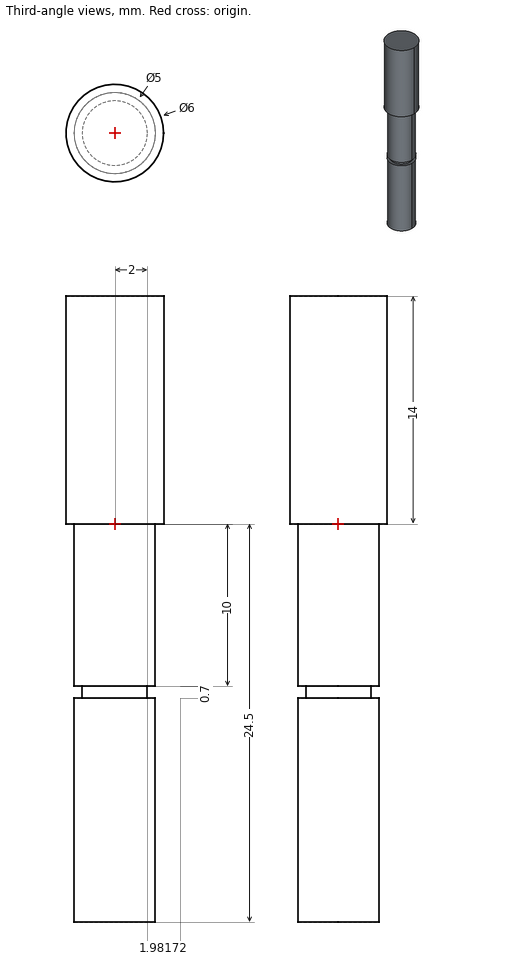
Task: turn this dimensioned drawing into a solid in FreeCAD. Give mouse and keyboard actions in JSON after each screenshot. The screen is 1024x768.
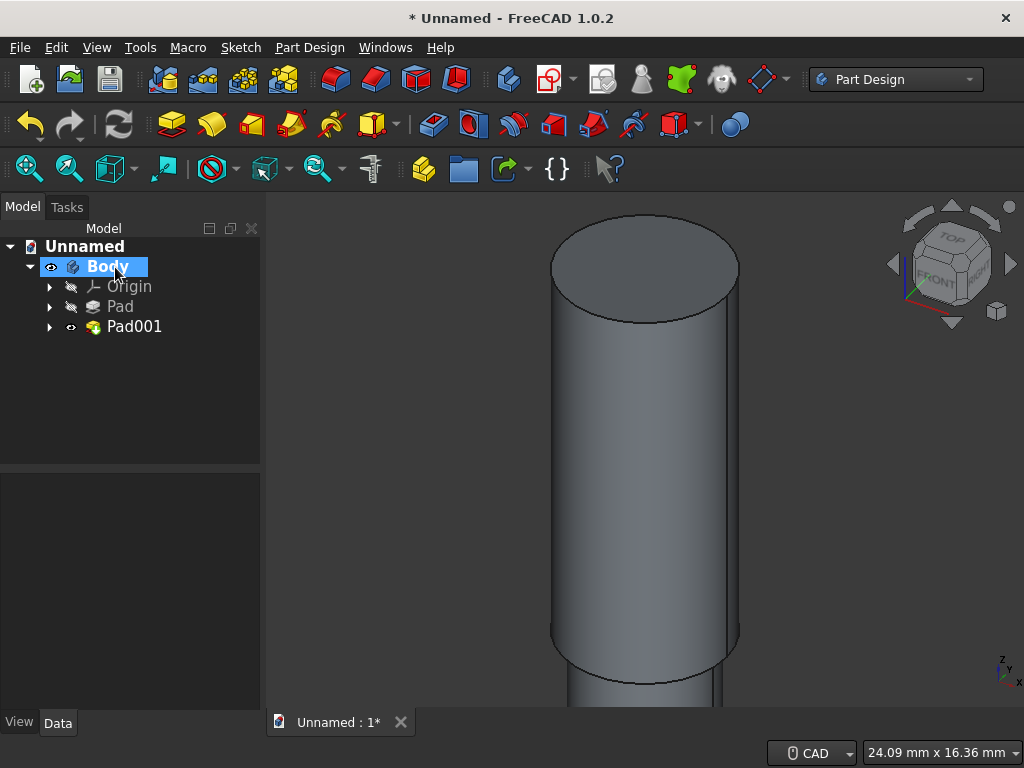
{"action": "left_click", "coordinate": [30, 170]}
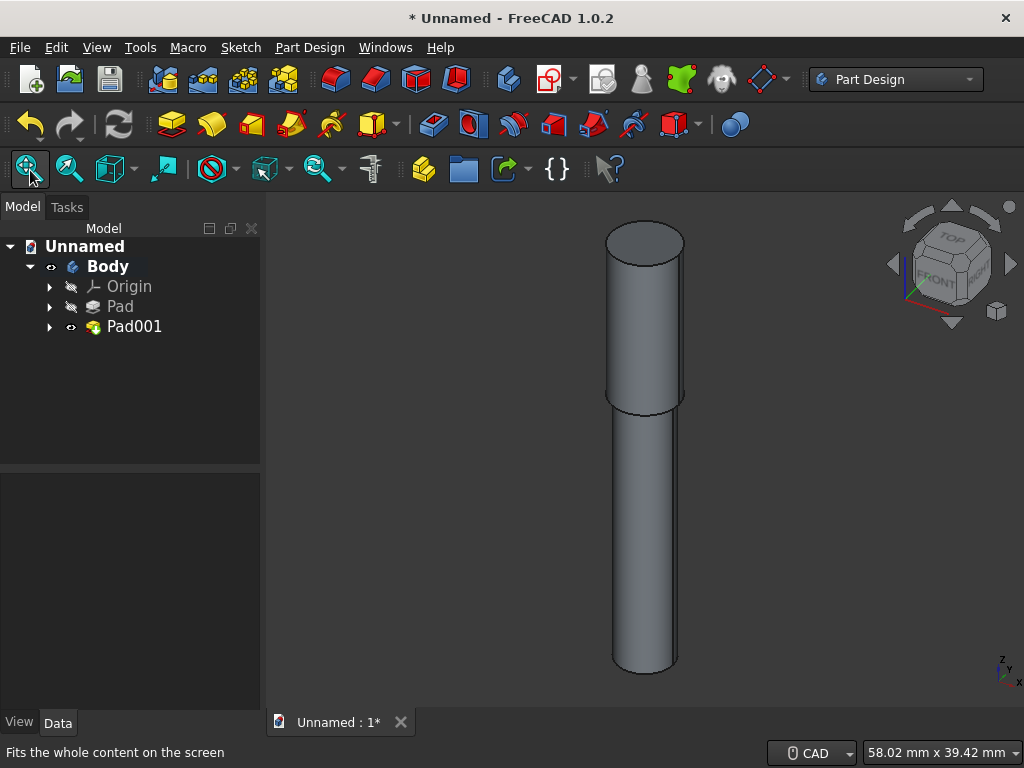
{"action": "left_click", "coordinate": [550, 80]}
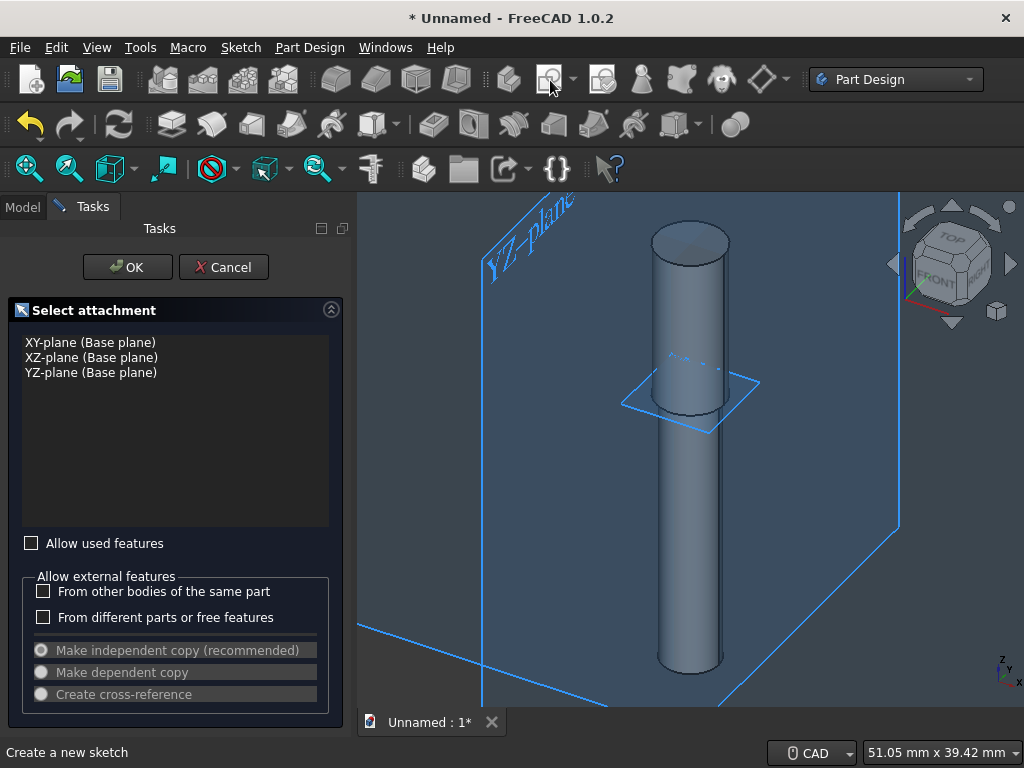
{"action": "left_click", "coordinate": [82, 358]}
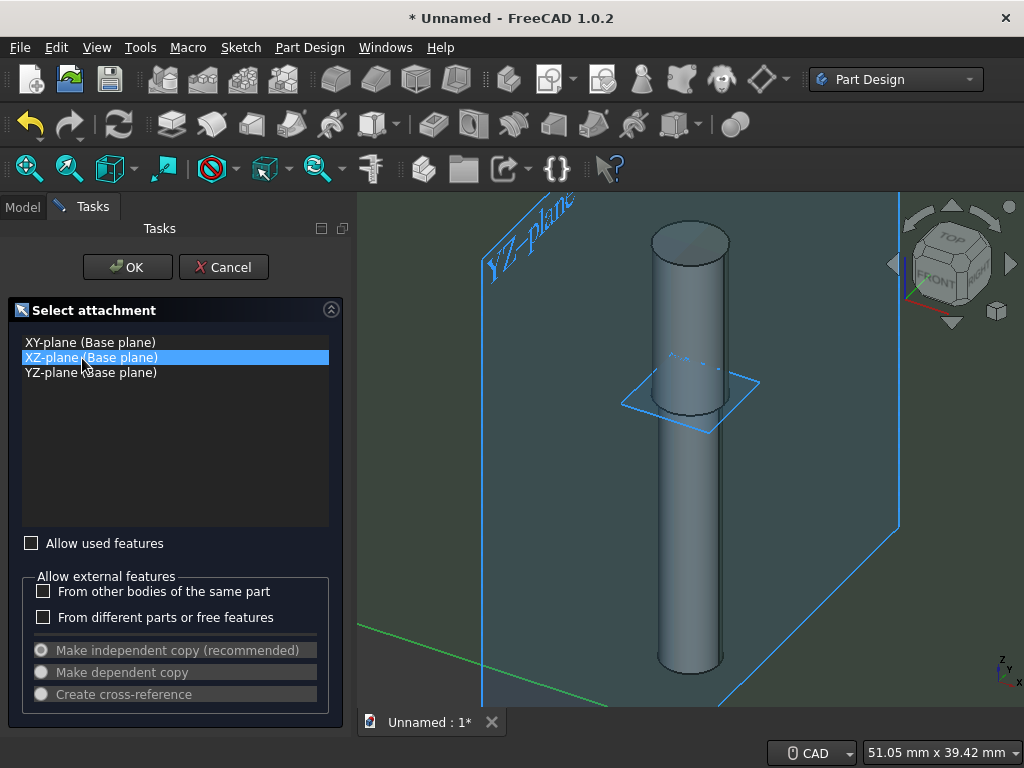
{"action": "left_click", "coordinate": [128, 267]}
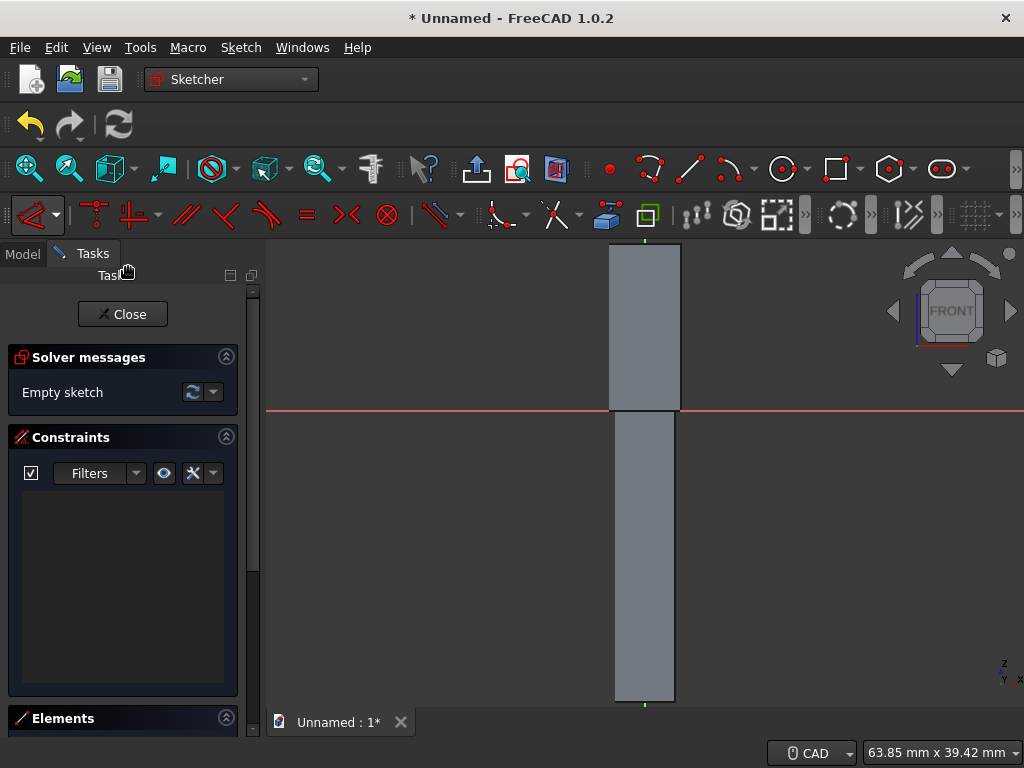
{"action": "left_click", "coordinate": [558, 170]}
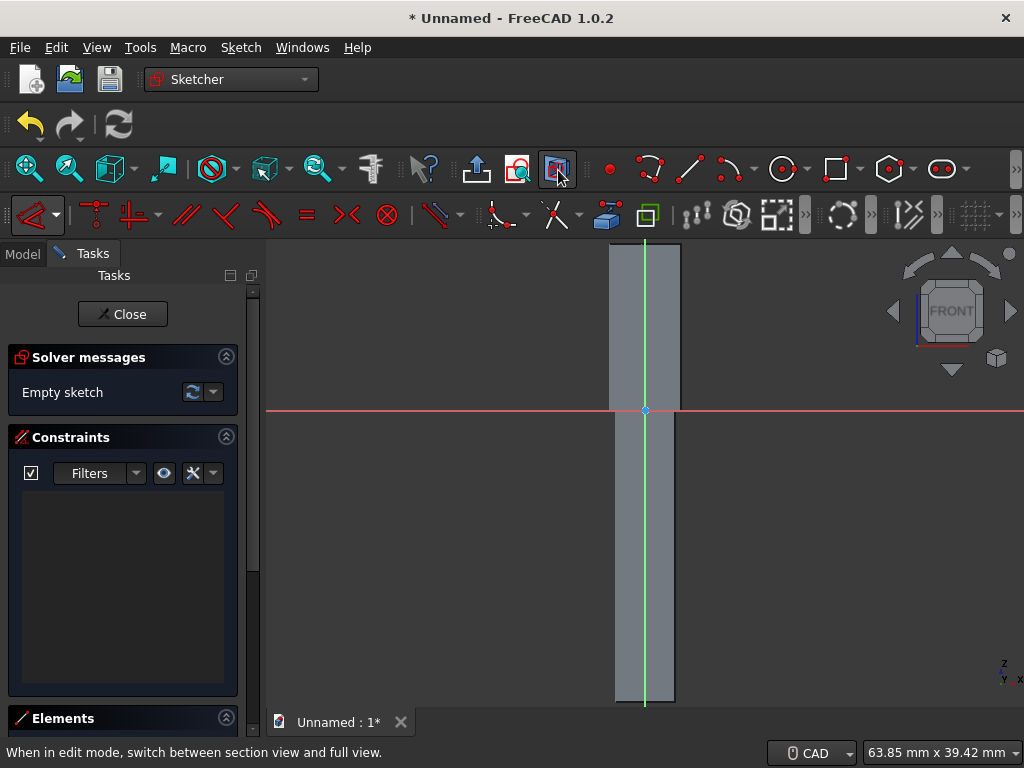
{"action": "scroll", "coordinate": [687, 537], "scroll_direction": "up", "scroll_amount": 14}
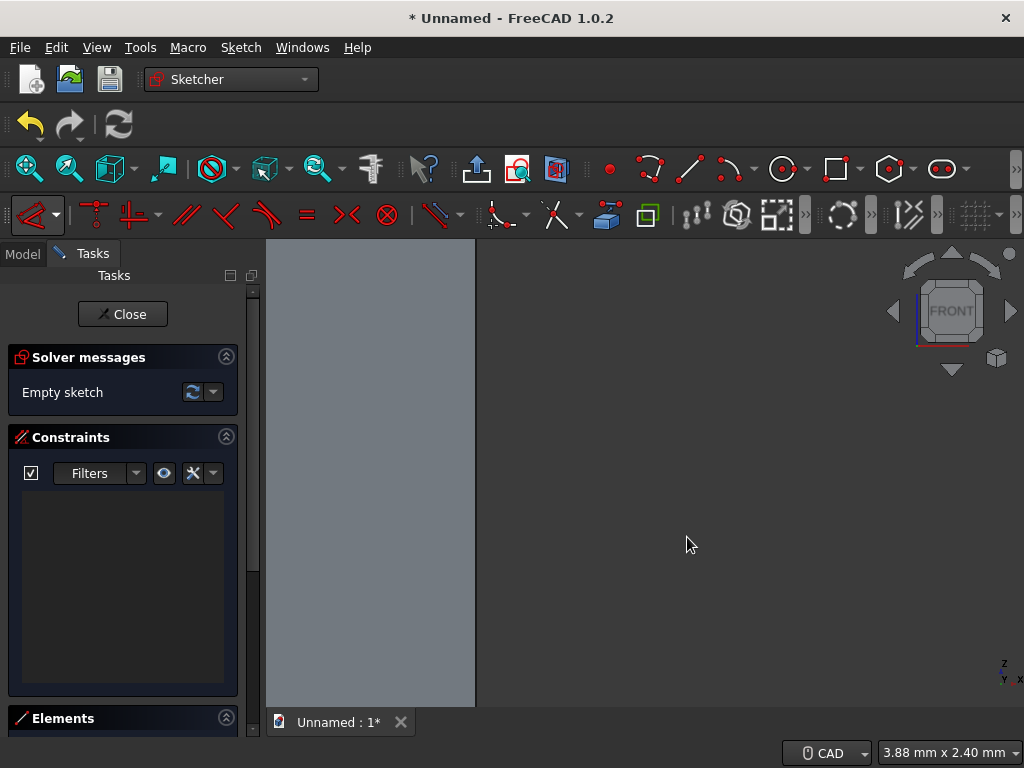
{"action": "left_click", "coordinate": [836, 170]}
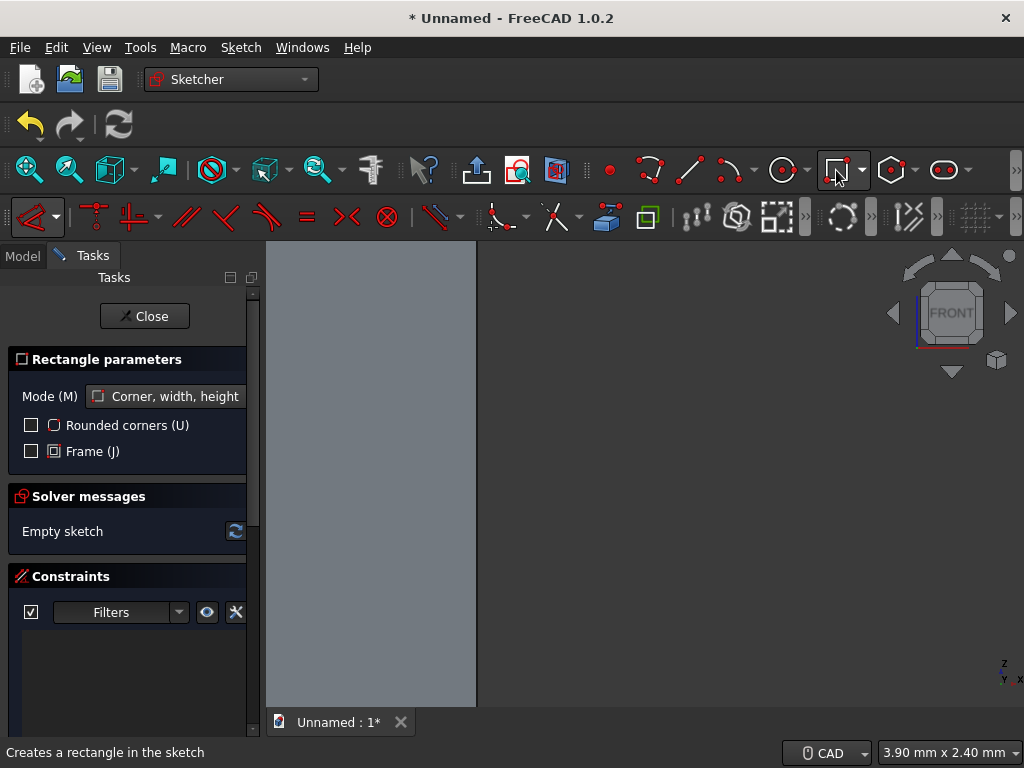
{"action": "left_click", "coordinate": [379, 403]}
{"action": "mouse_move", "coordinate": [765, 539]}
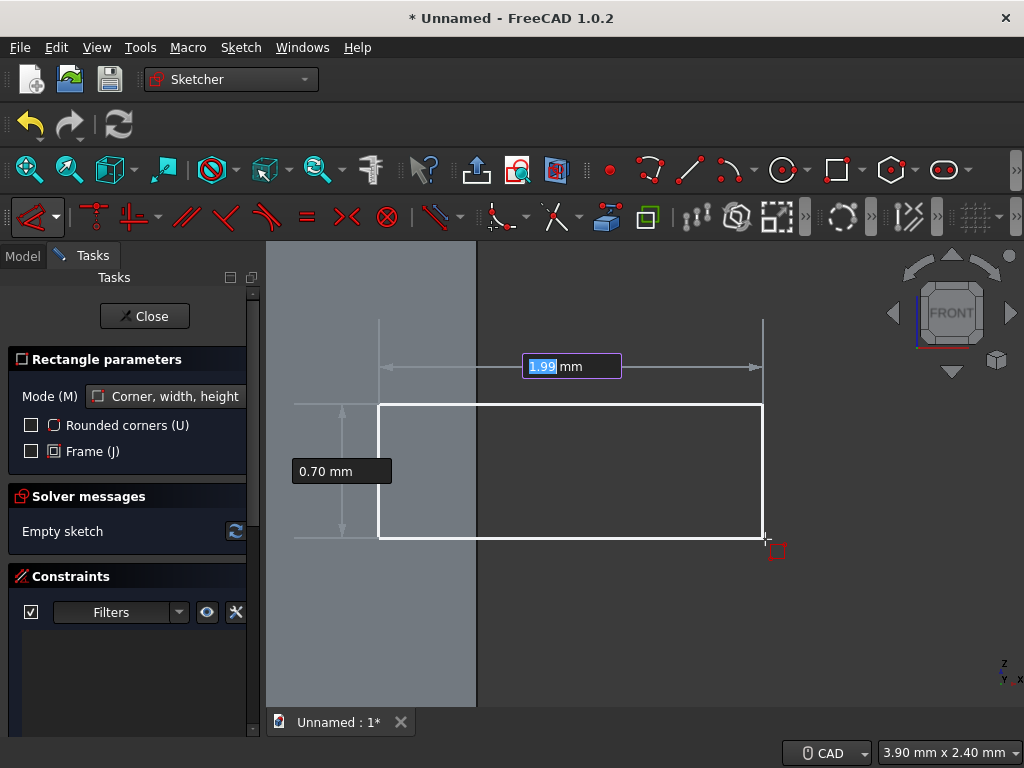
{"action": "type", "text": "1.98172"}
{"action": "key", "text": "Tab"}
{"action": "type", "text": "0.7"}
{"action": "key", "text": "Return"}
{"action": "key", "text": "Escape"}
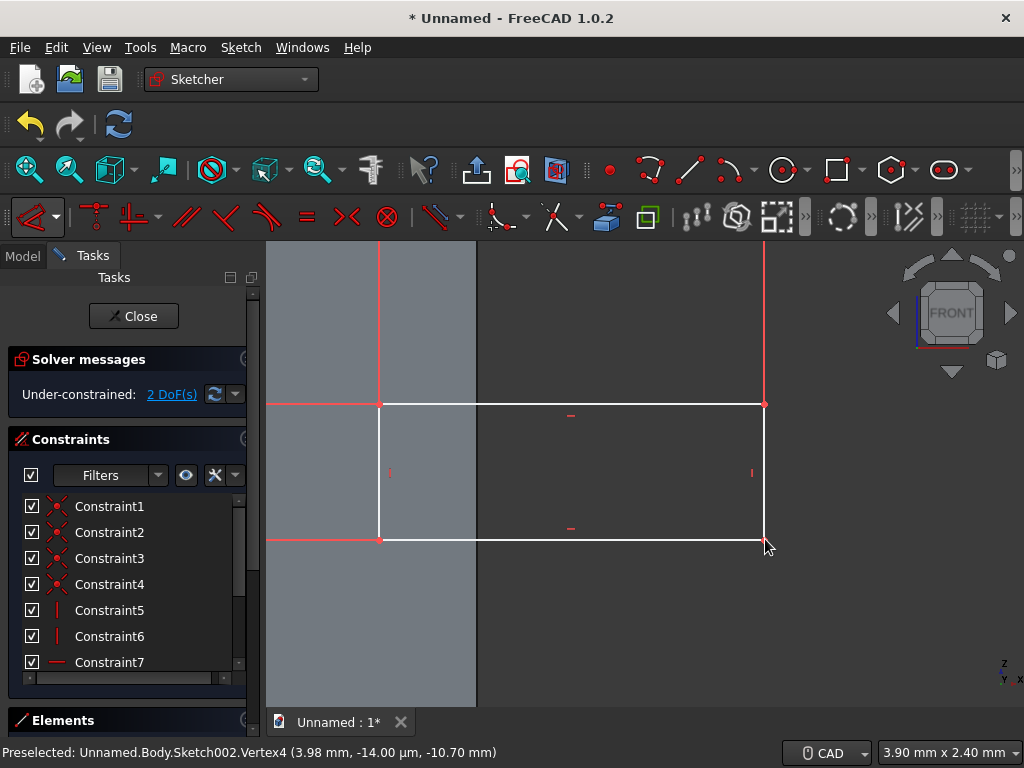
{"action": "left_click", "coordinate": [32, 218]}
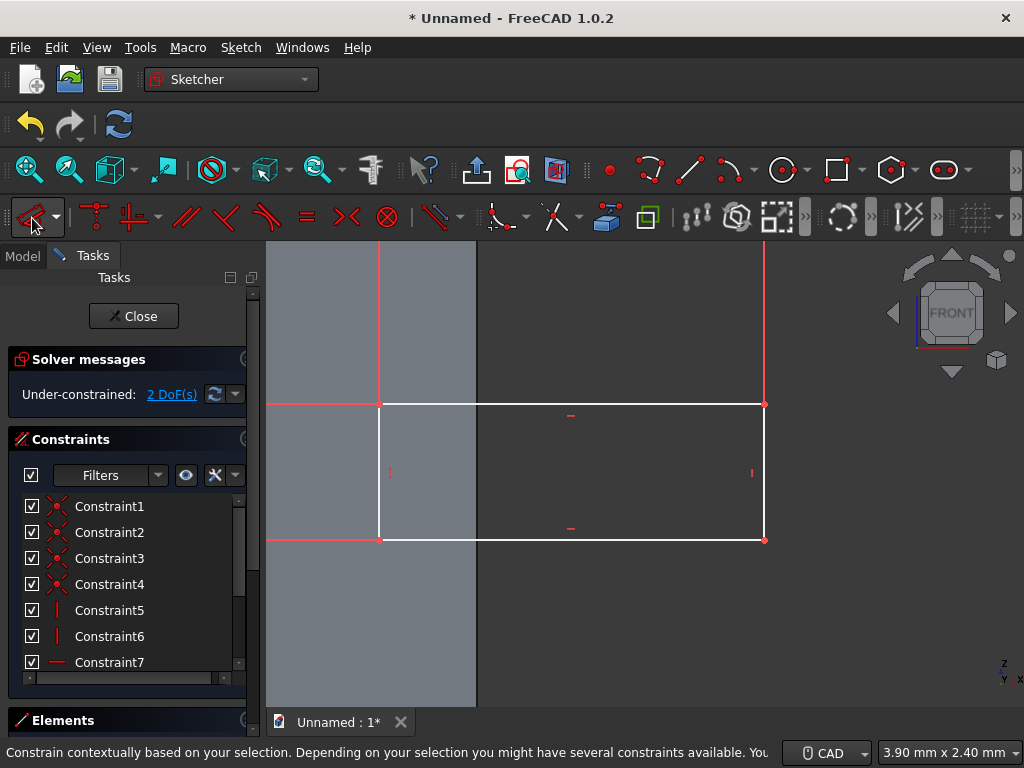
{"action": "left_click", "coordinate": [379, 404]}
{"action": "left_click", "coordinate": [336, 438]}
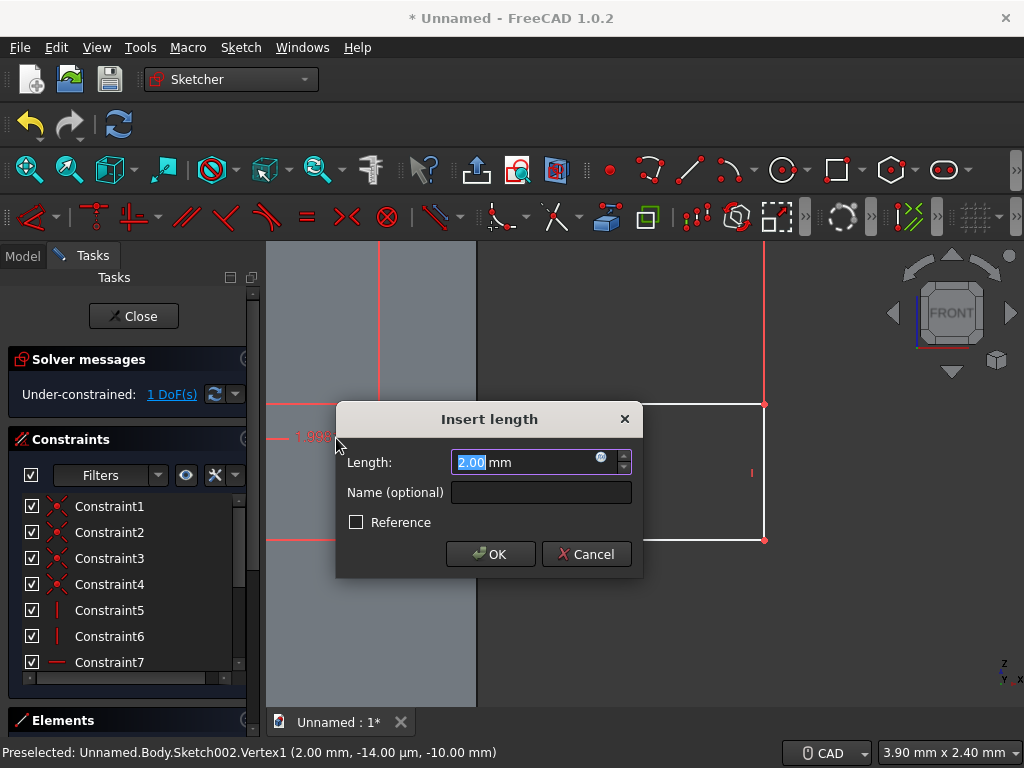
{"action": "type", "text": "2"}
{"action": "key", "text": "Return"}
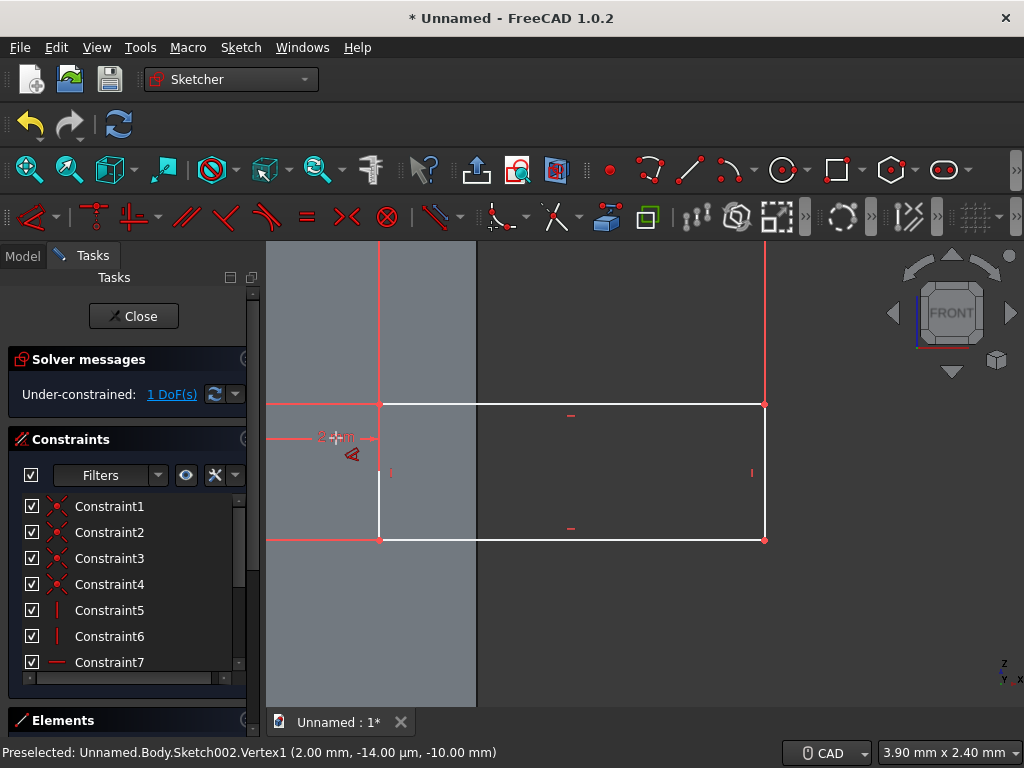
{"action": "left_click", "coordinate": [379, 404]}
{"action": "left_click", "coordinate": [413, 336]}